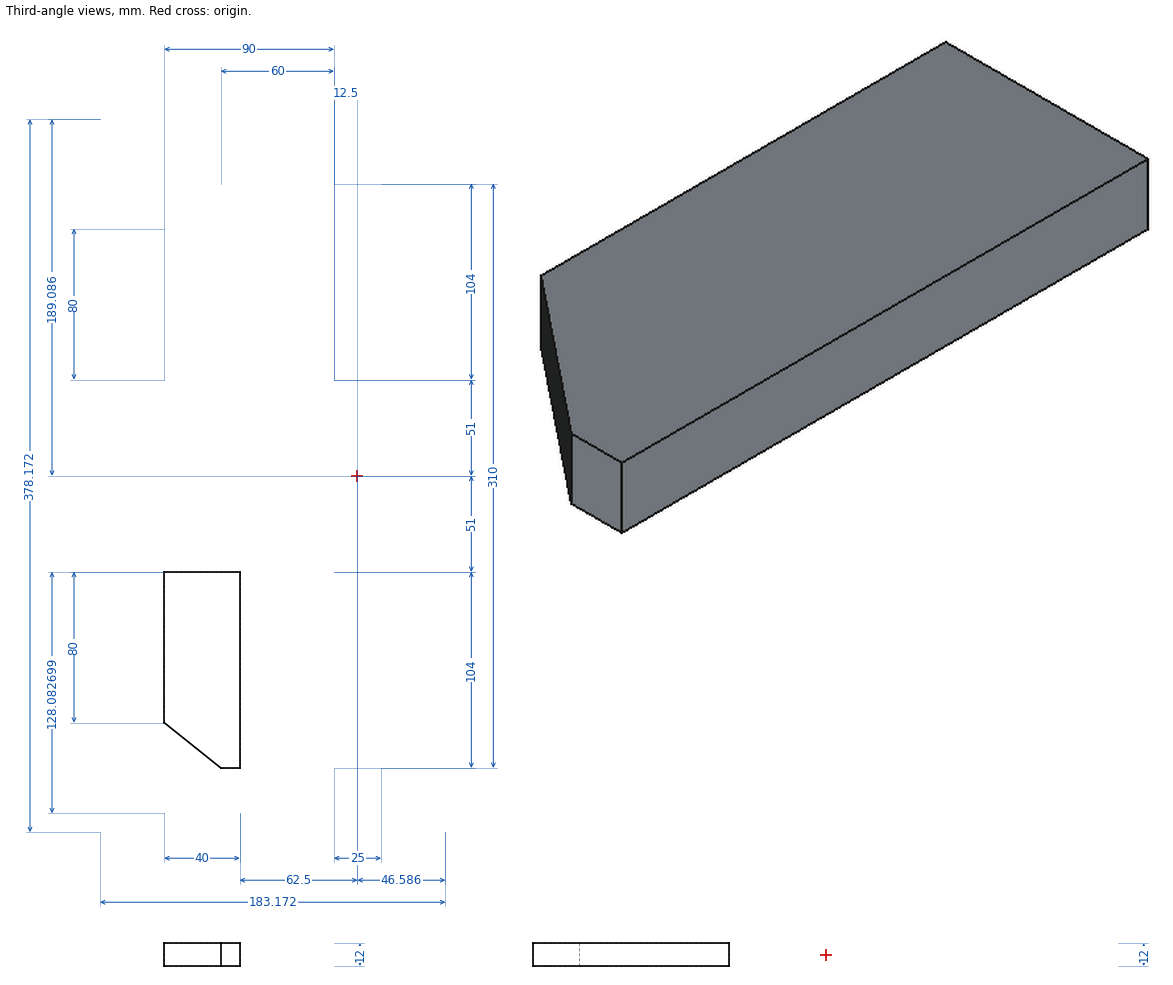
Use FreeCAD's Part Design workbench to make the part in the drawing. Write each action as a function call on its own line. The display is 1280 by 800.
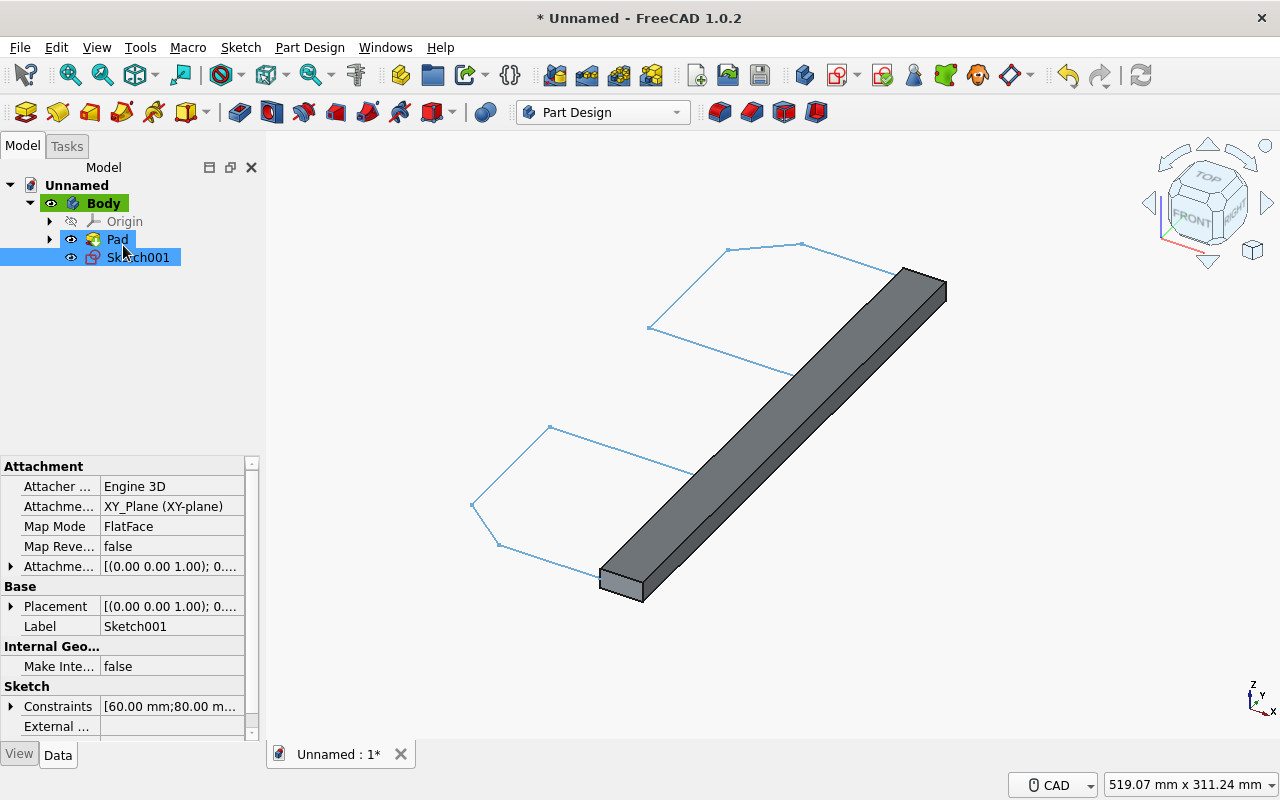
click(26, 112)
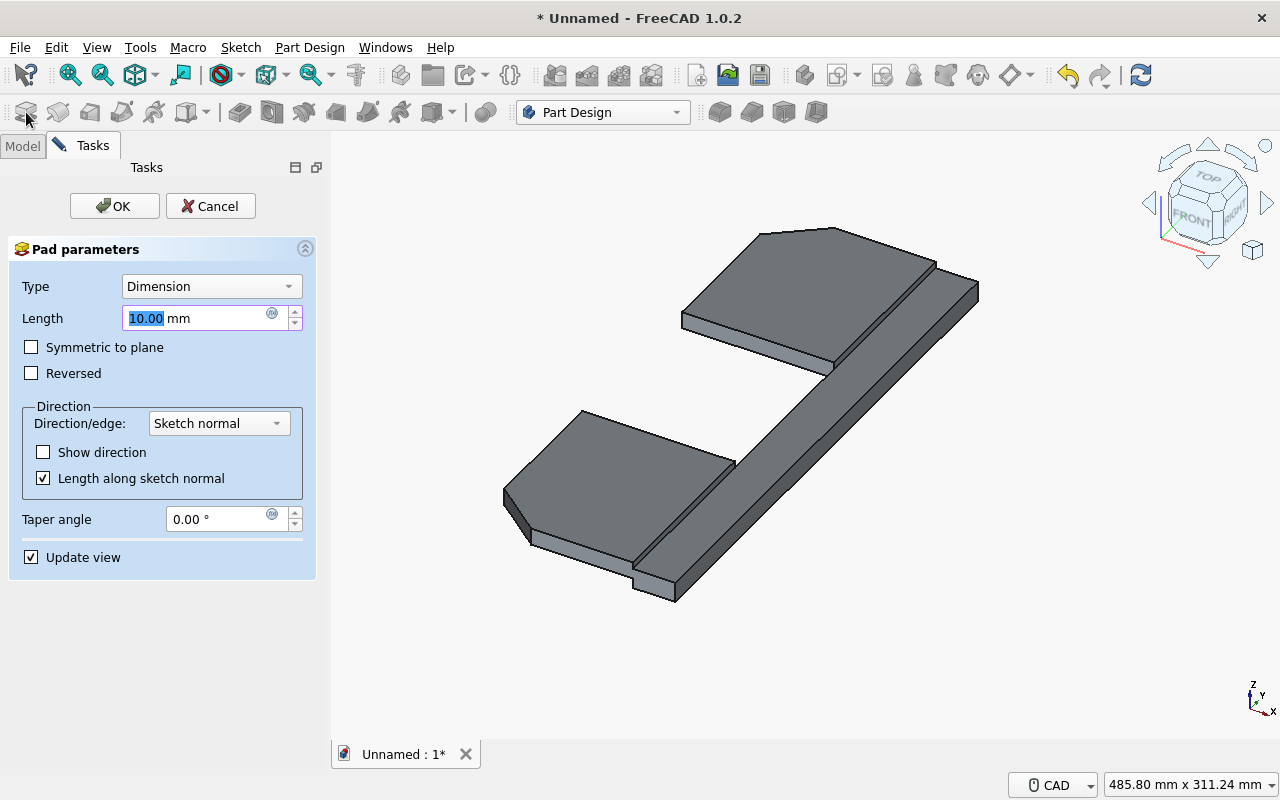
text(12)
key(Tab)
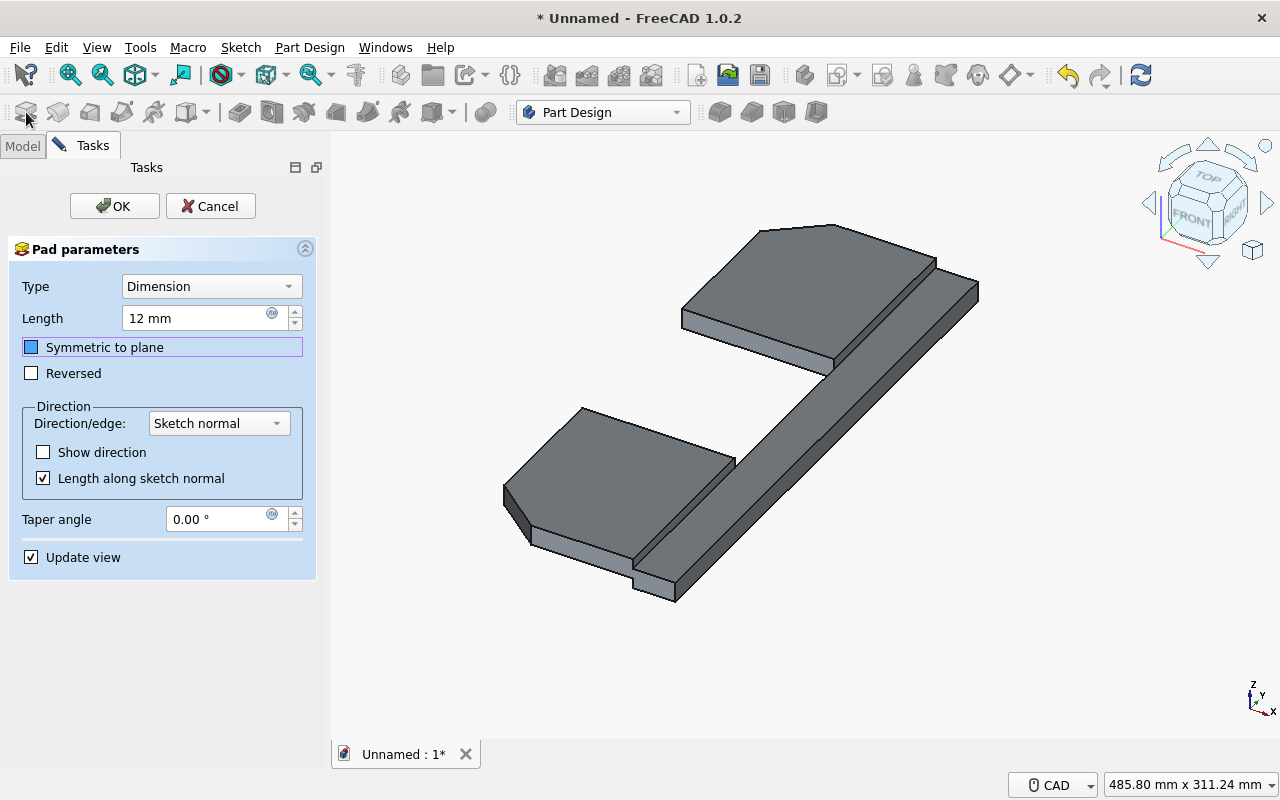
click(30, 347)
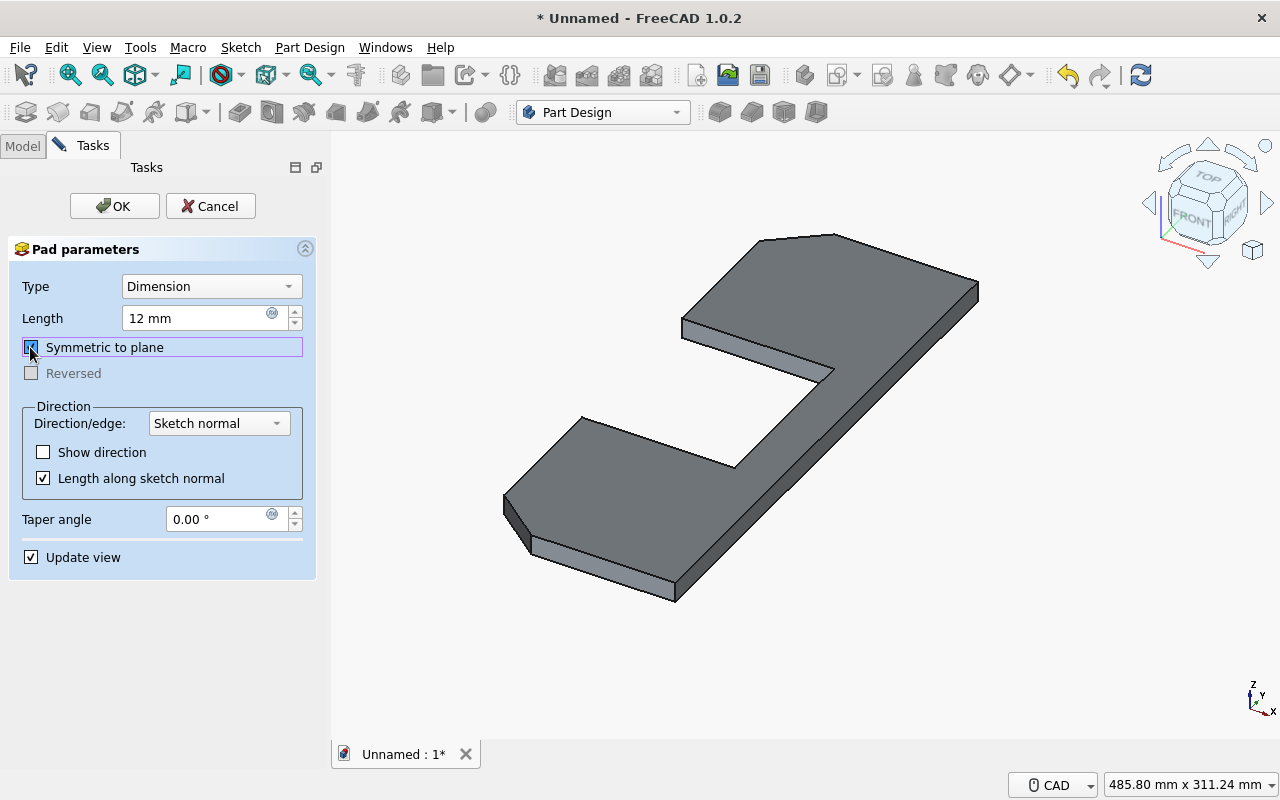
click(115, 206)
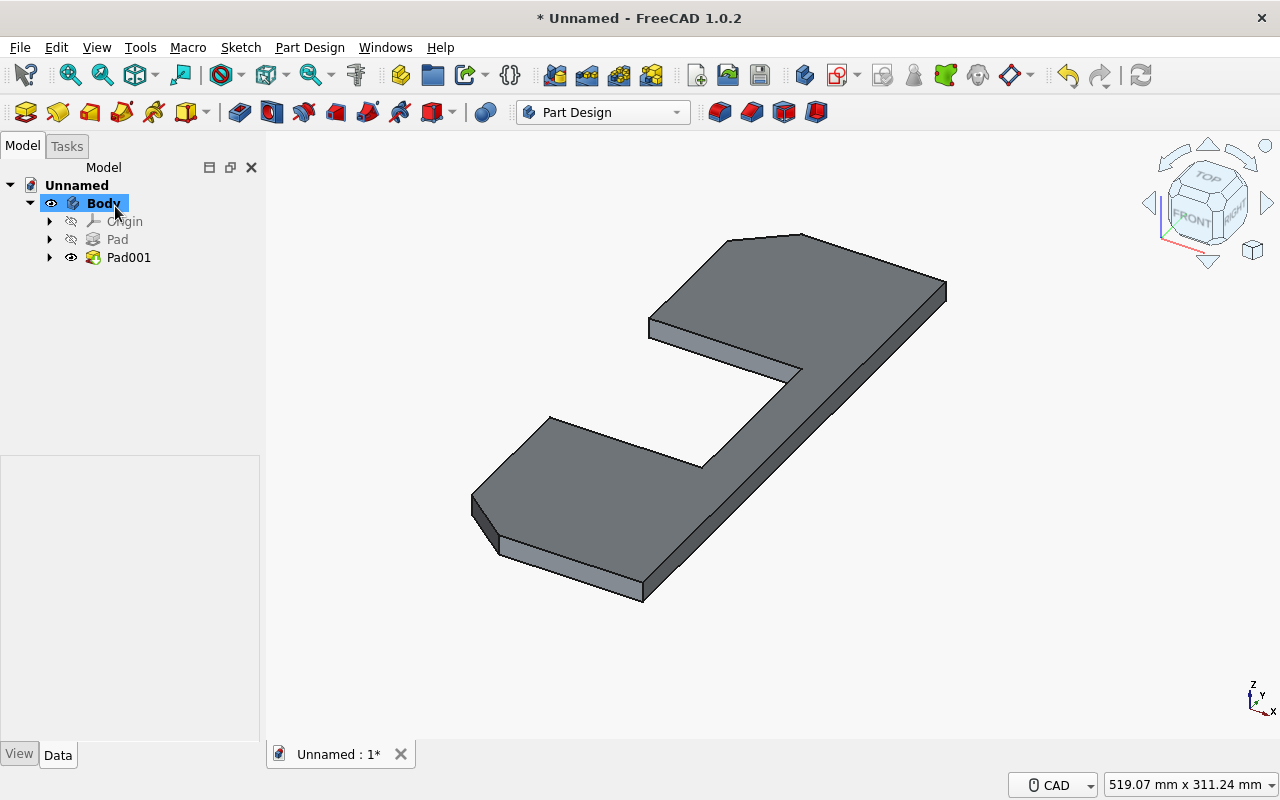
click(811, 322)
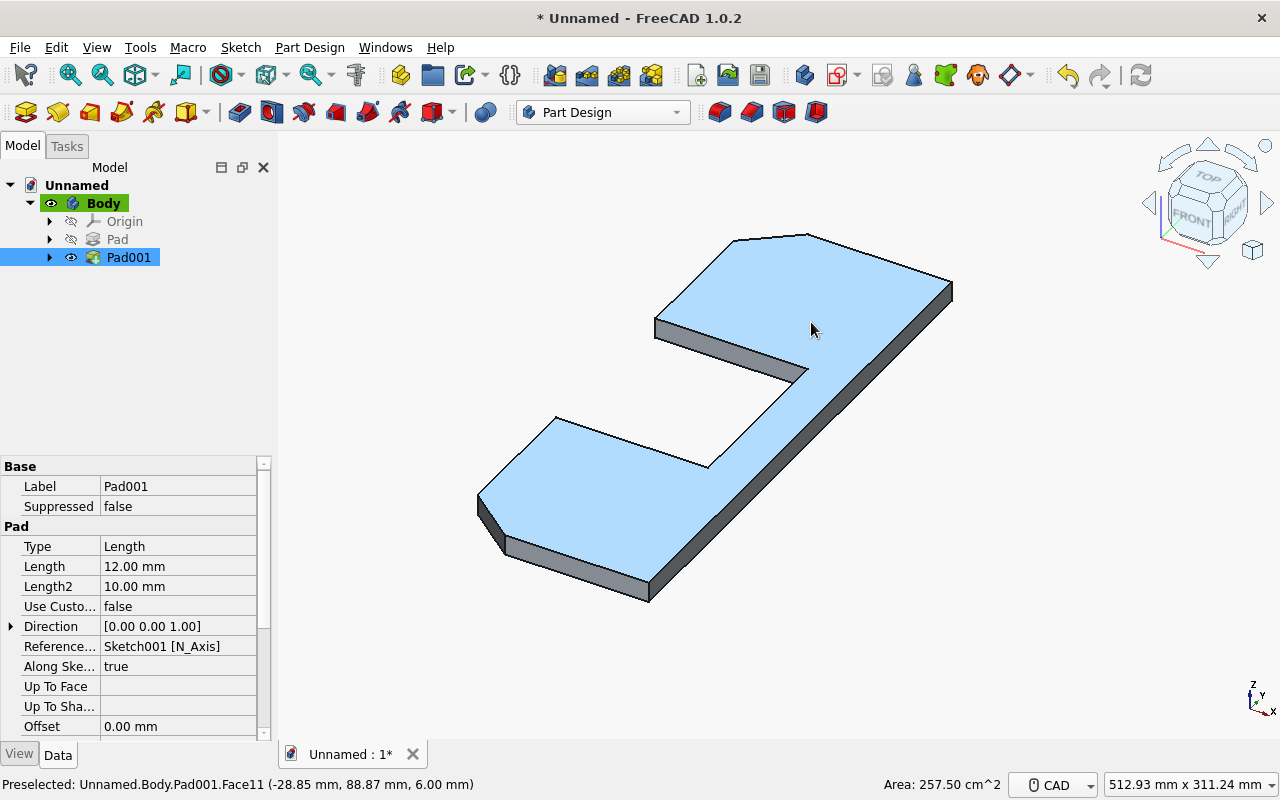
click(838, 76)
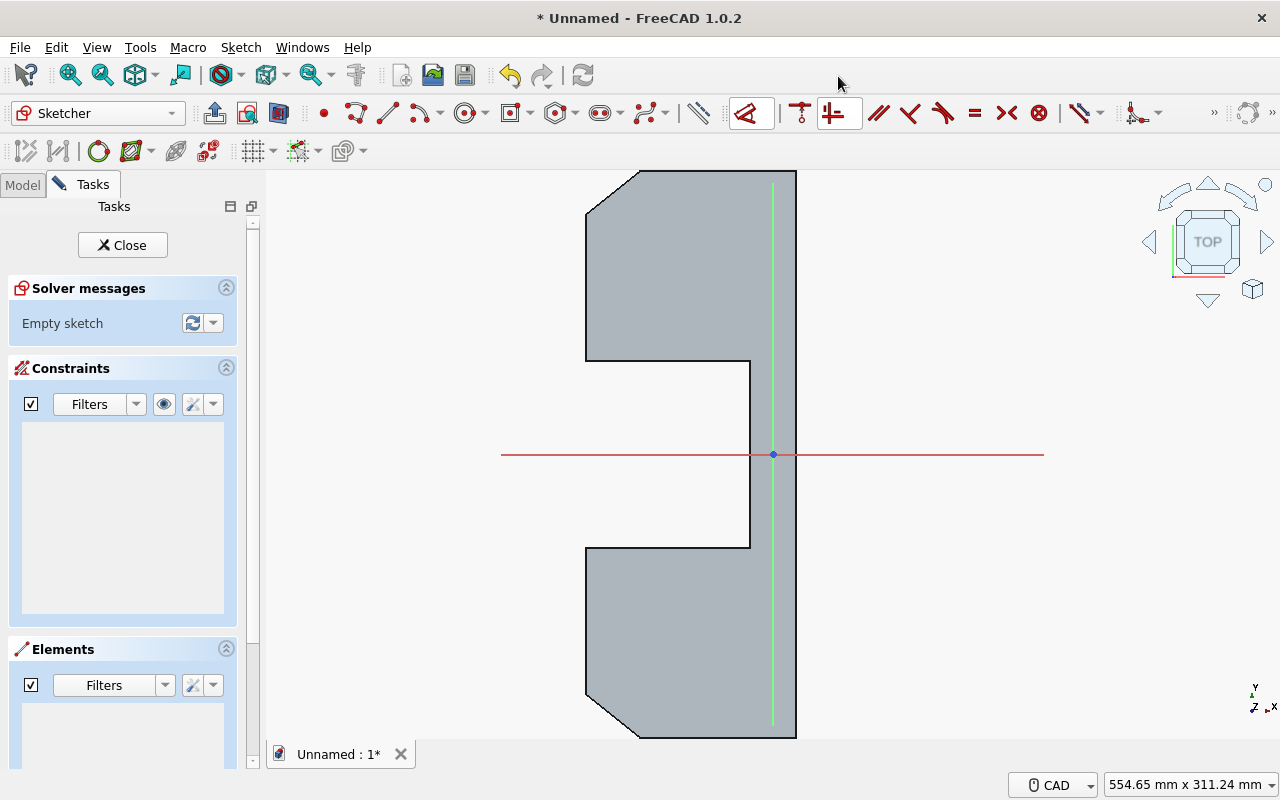
scroll(721, 454, down, 3)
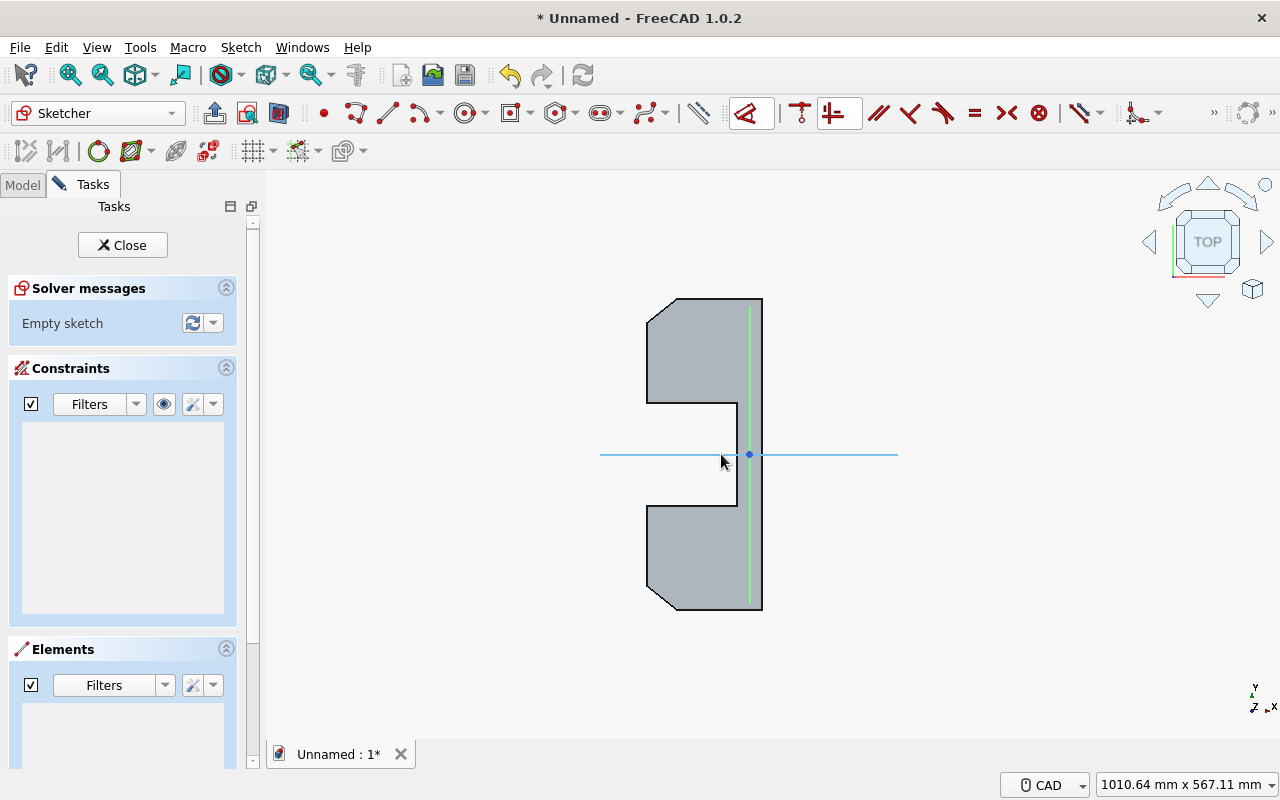
click(532, 114)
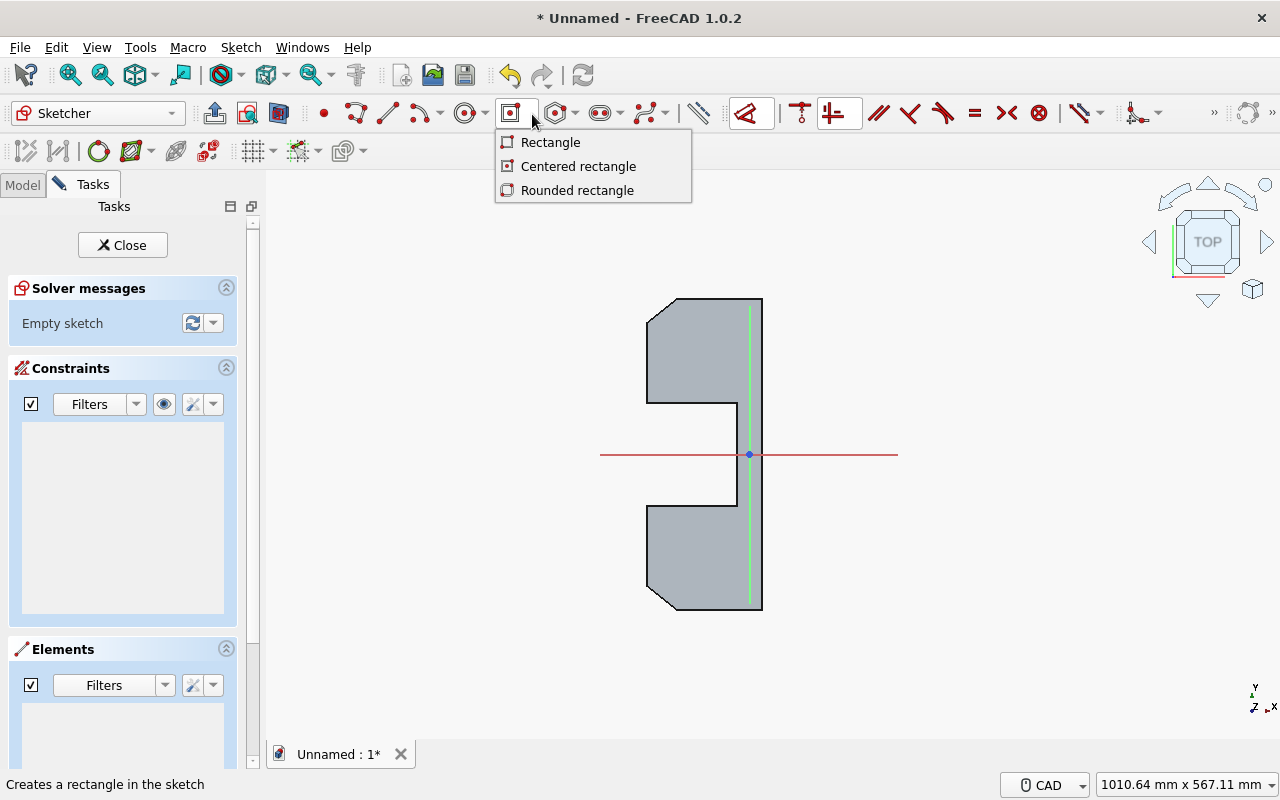
click(594, 142)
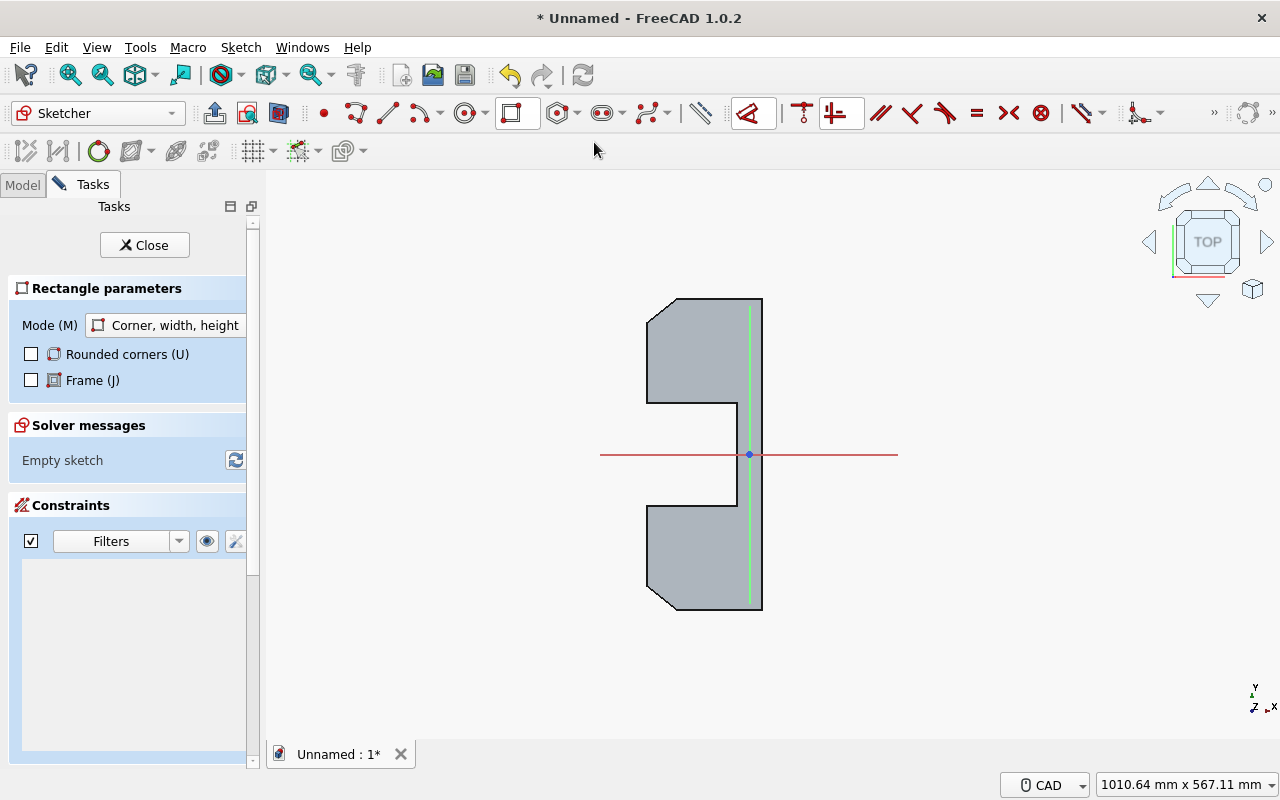
click(613, 265)
click(796, 644)